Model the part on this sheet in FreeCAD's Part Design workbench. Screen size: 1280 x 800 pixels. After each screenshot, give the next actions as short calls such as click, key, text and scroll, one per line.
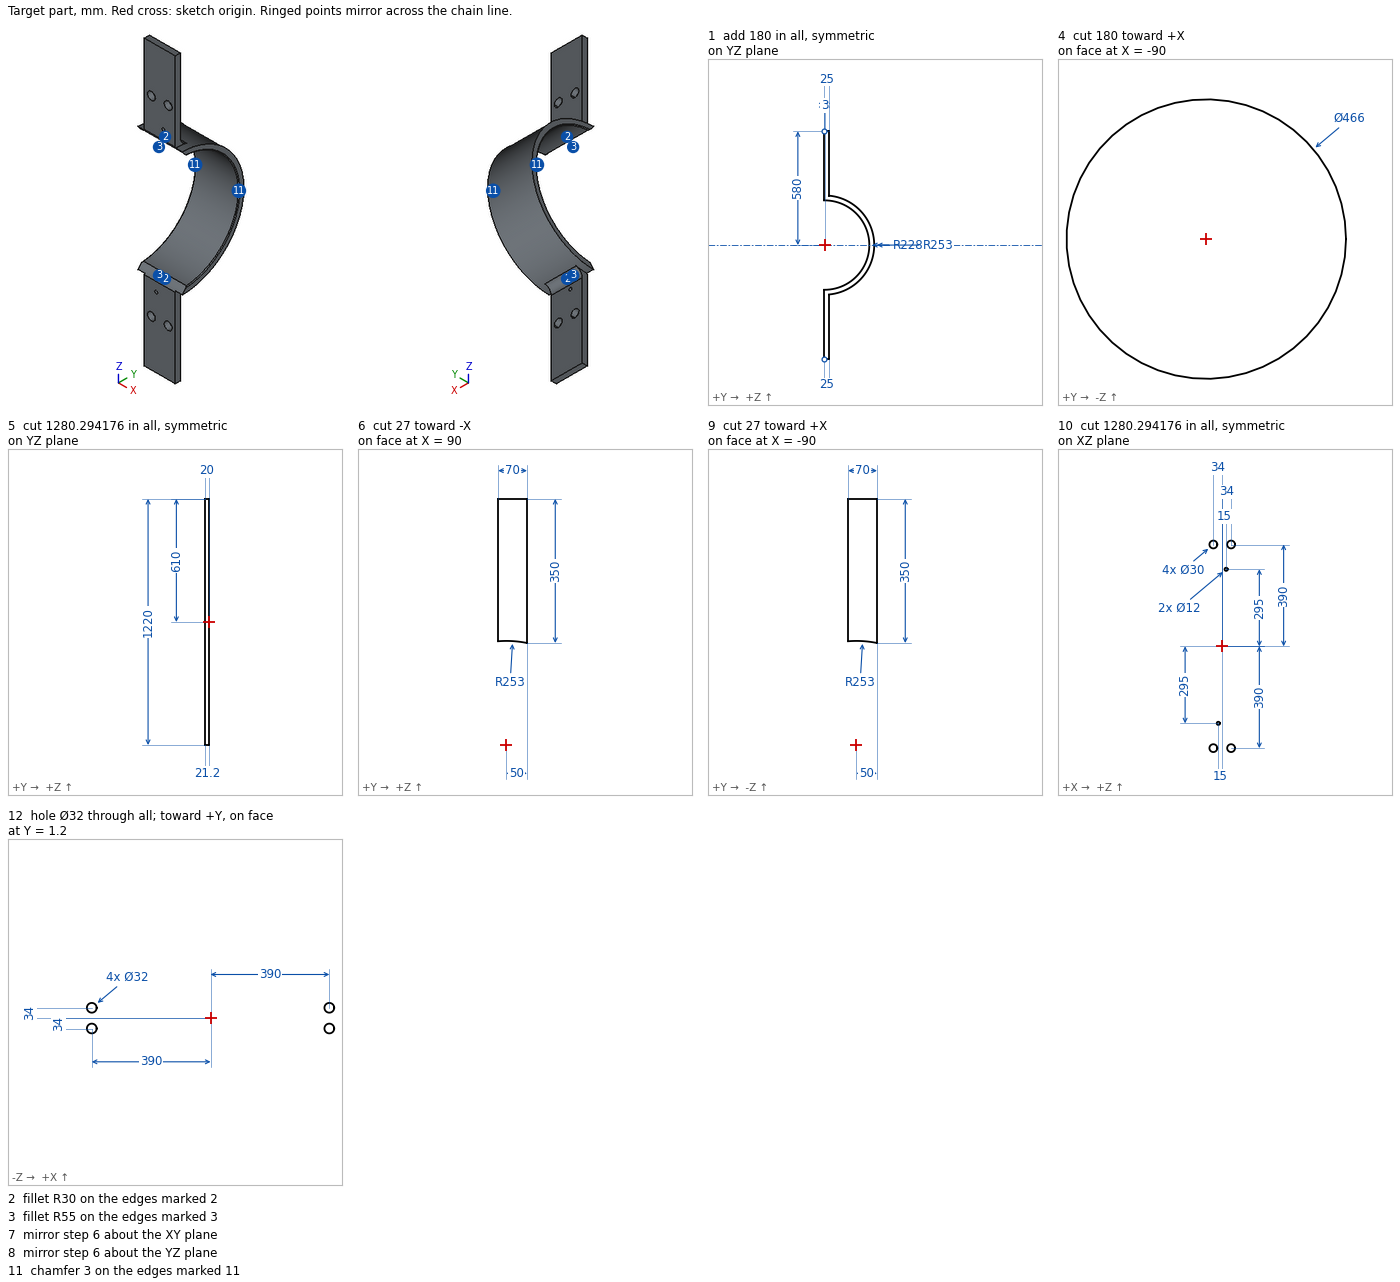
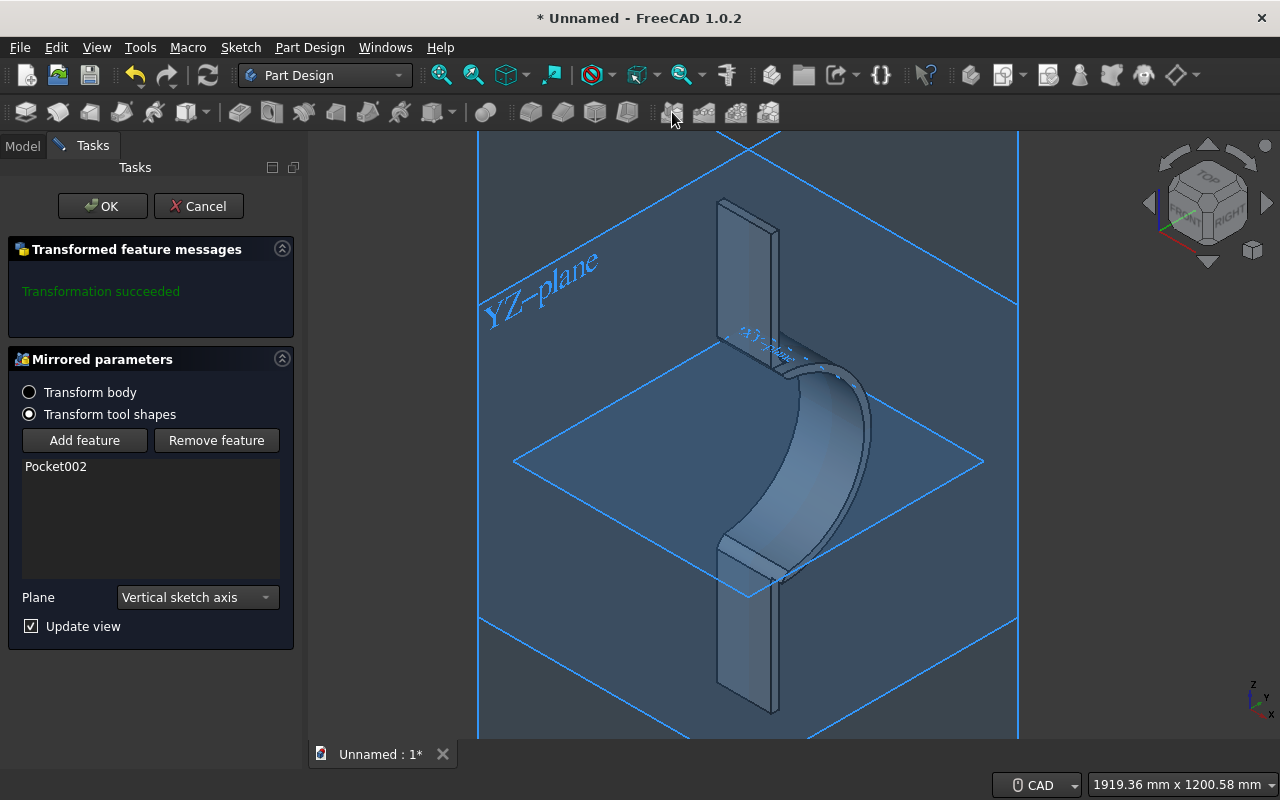
click(198, 598)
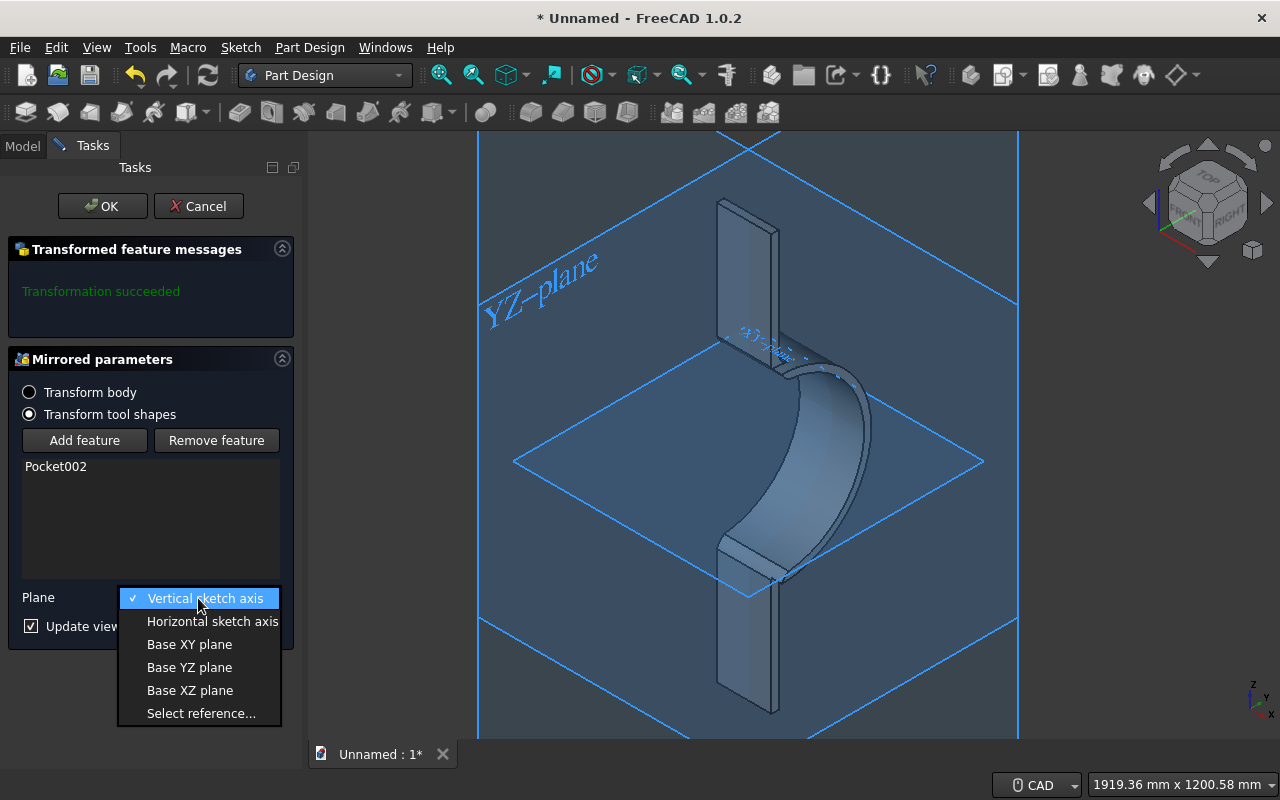
click(198, 668)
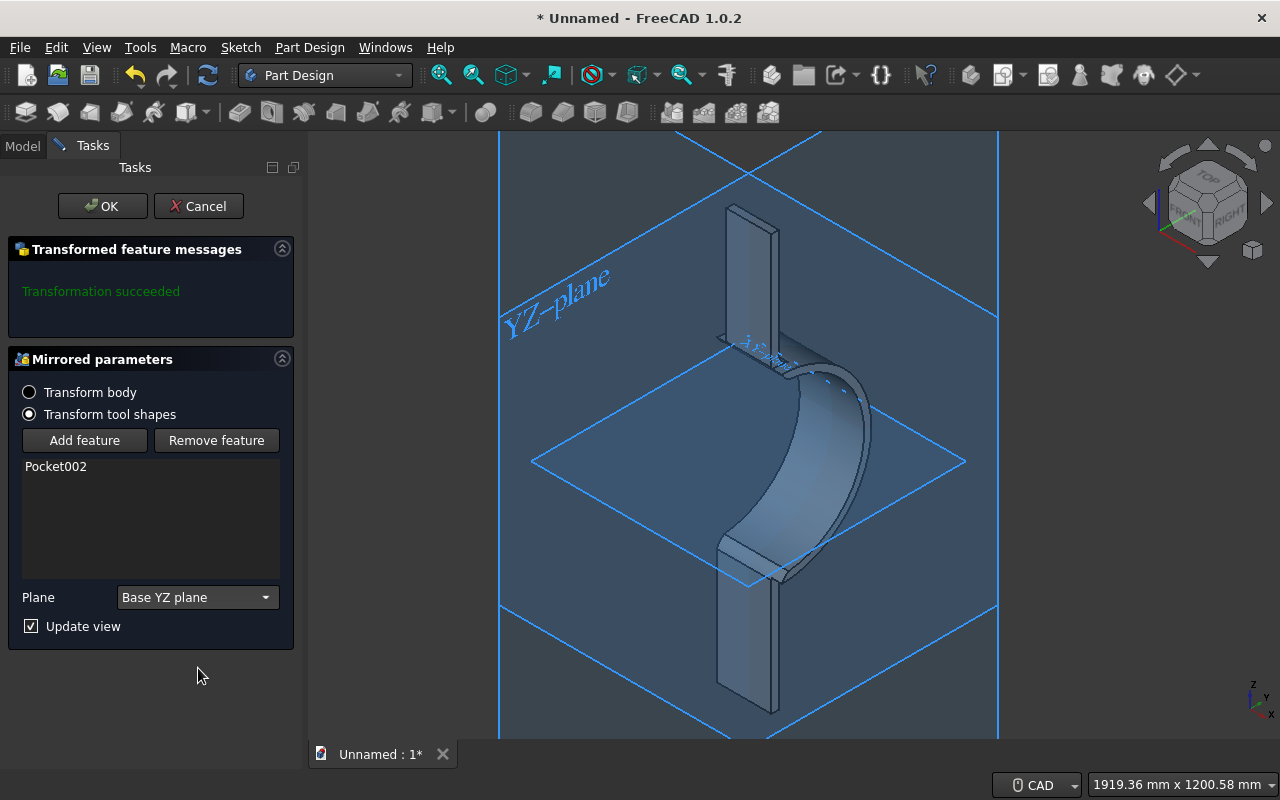
click(103, 206)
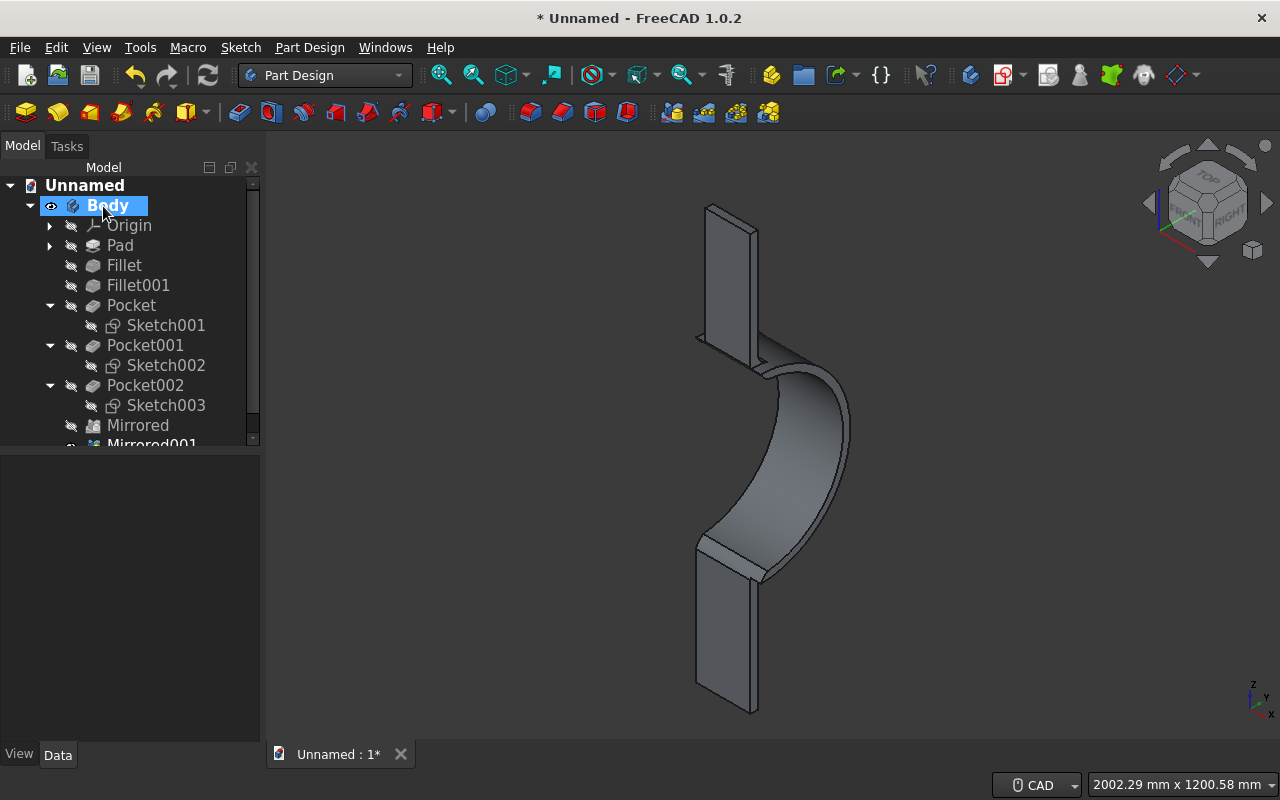
key(6)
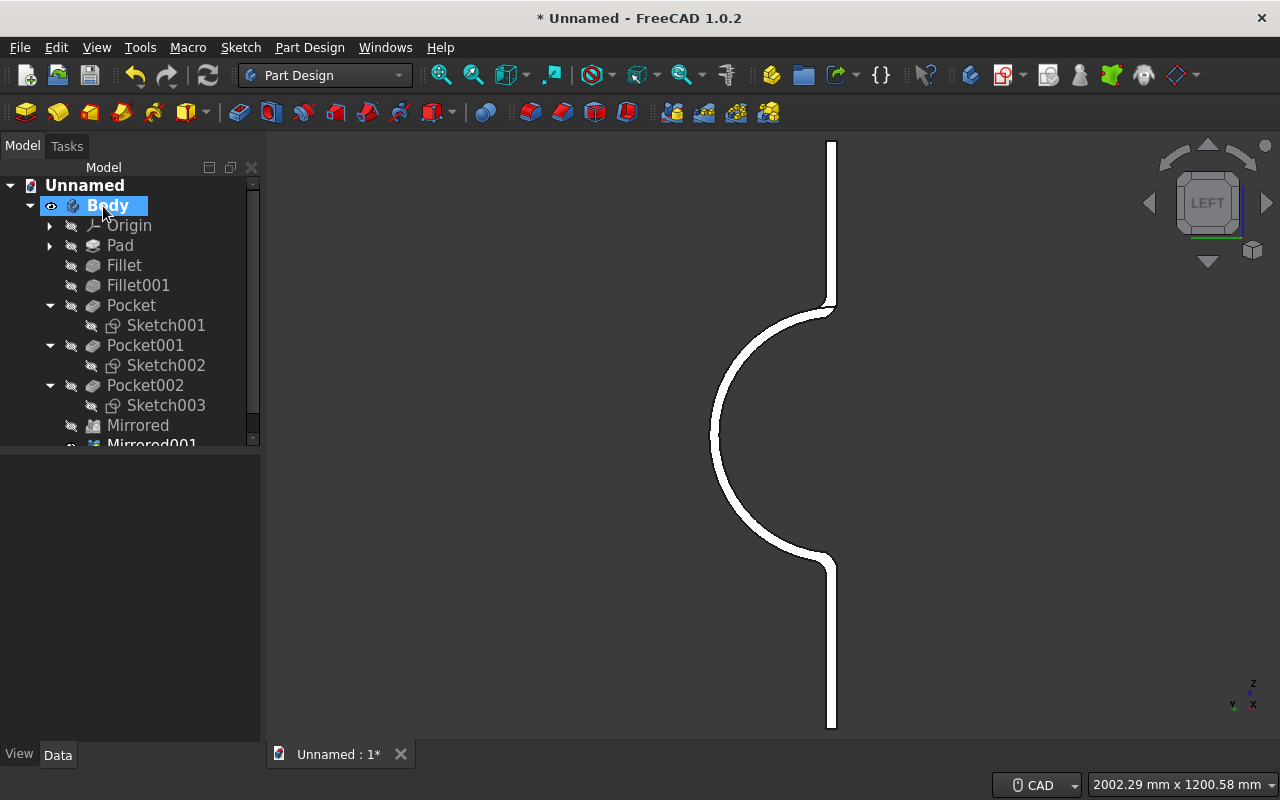
scroll(718, 396, up, 7)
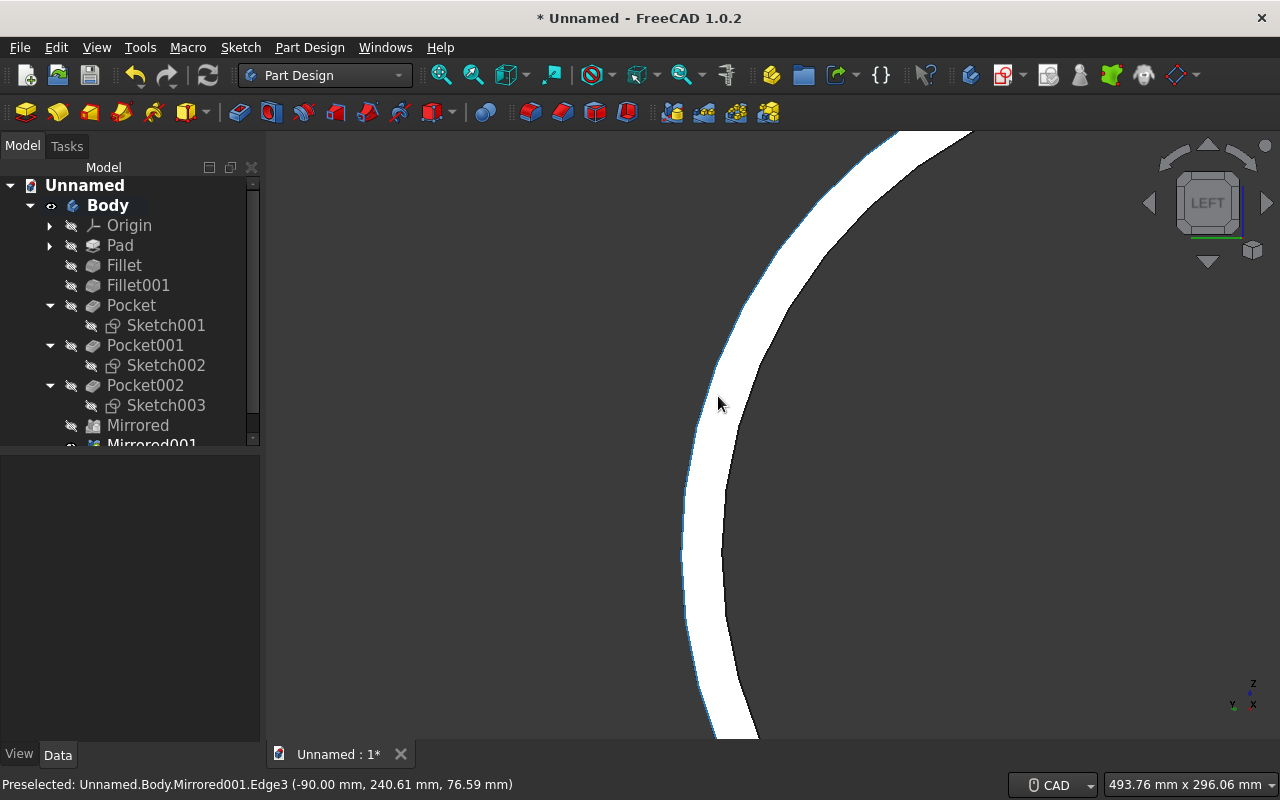
click(718, 399)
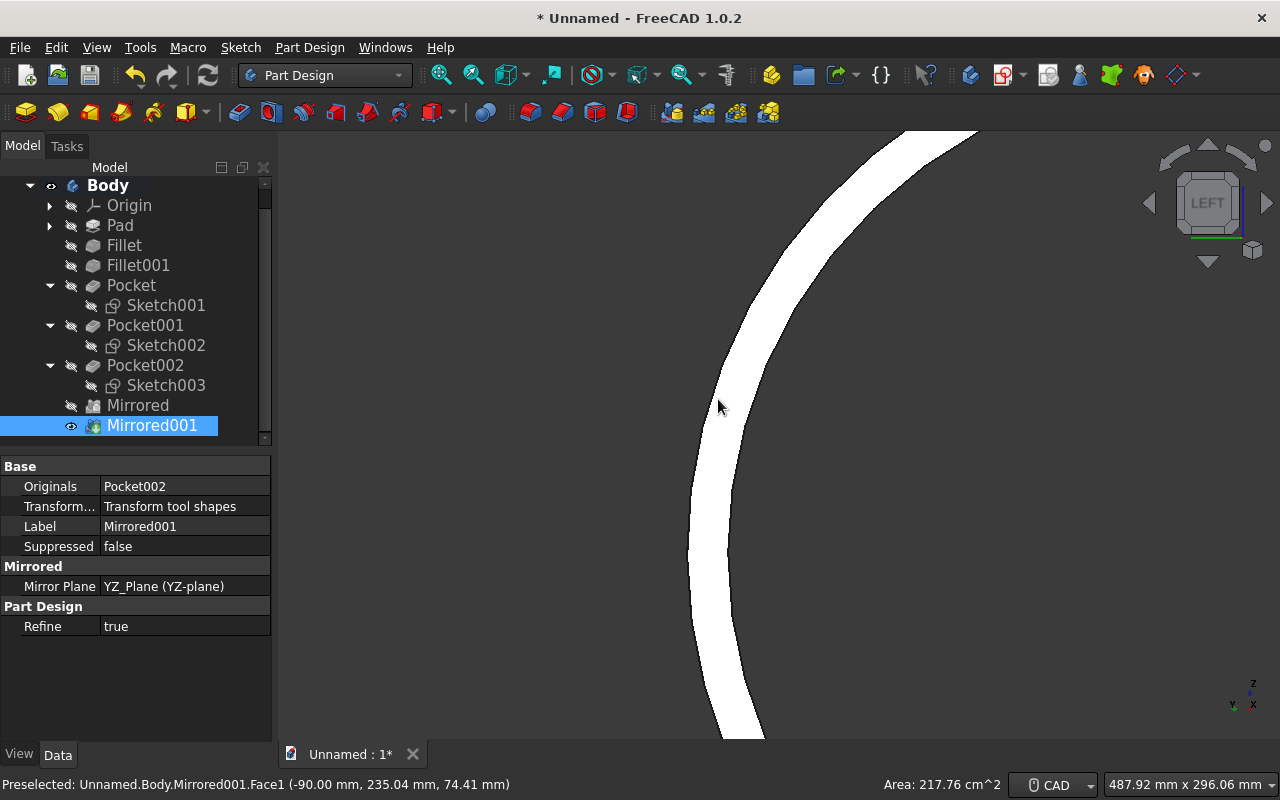
click(1004, 76)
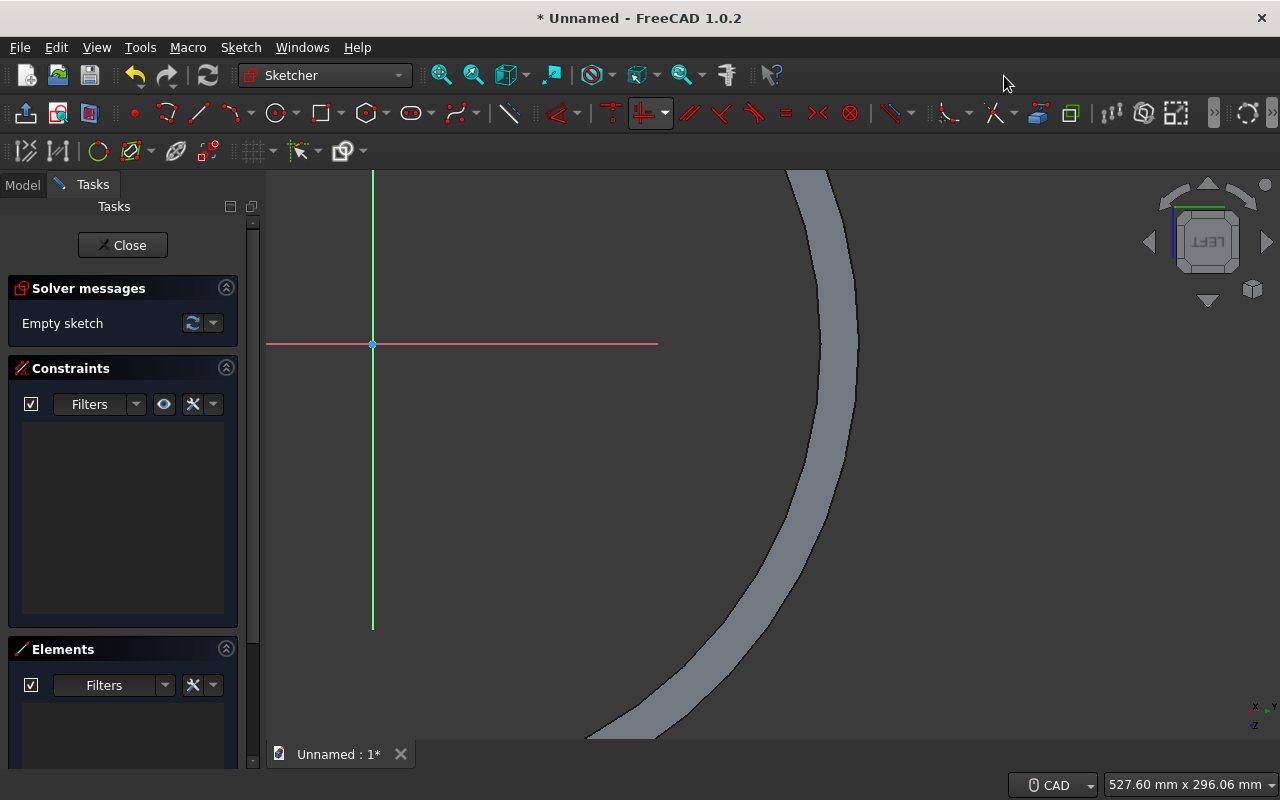
scroll(835, 711, down, 6)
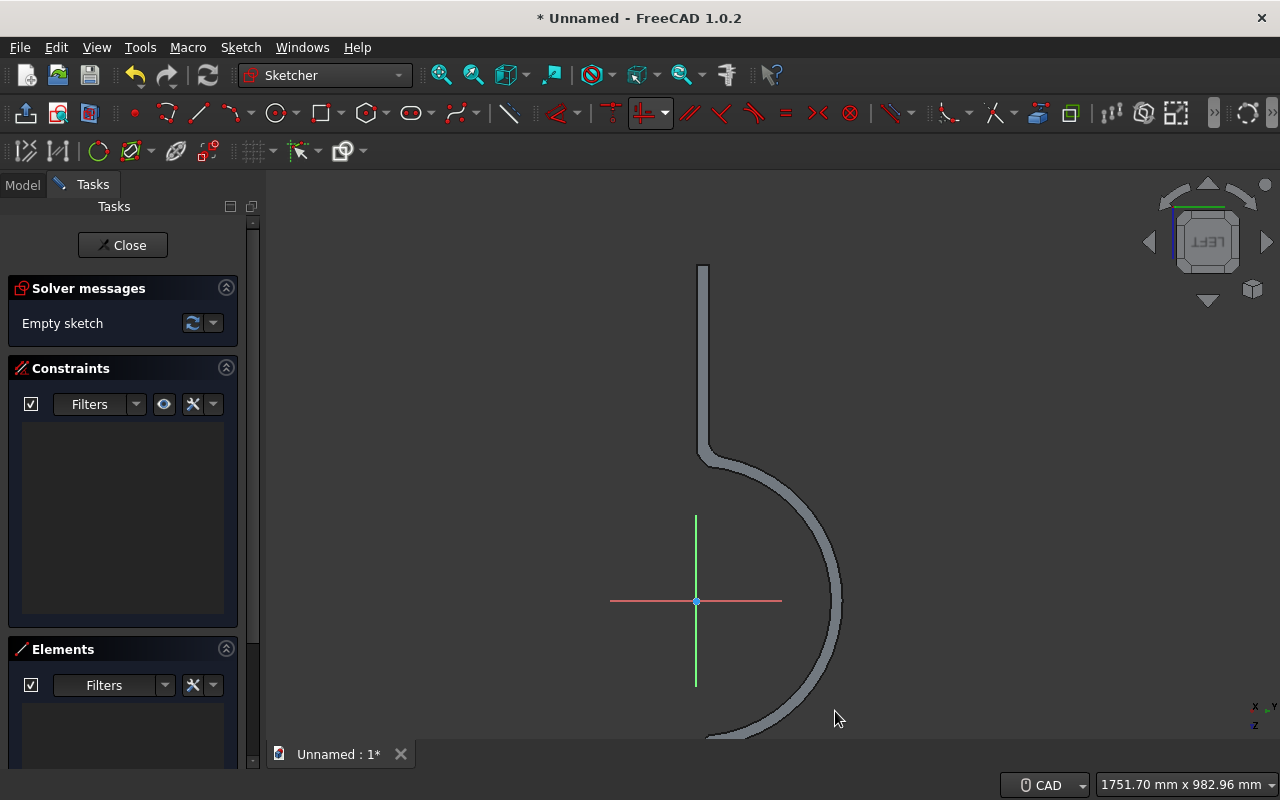
click(168, 114)